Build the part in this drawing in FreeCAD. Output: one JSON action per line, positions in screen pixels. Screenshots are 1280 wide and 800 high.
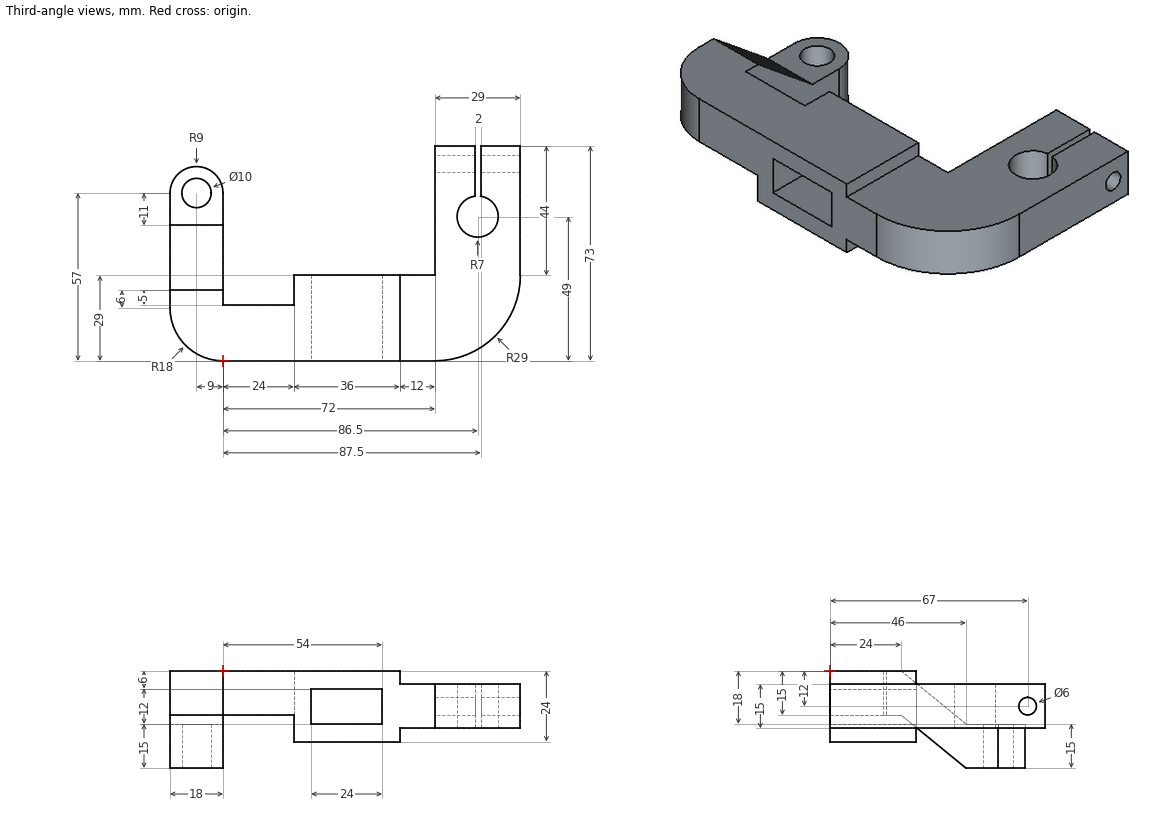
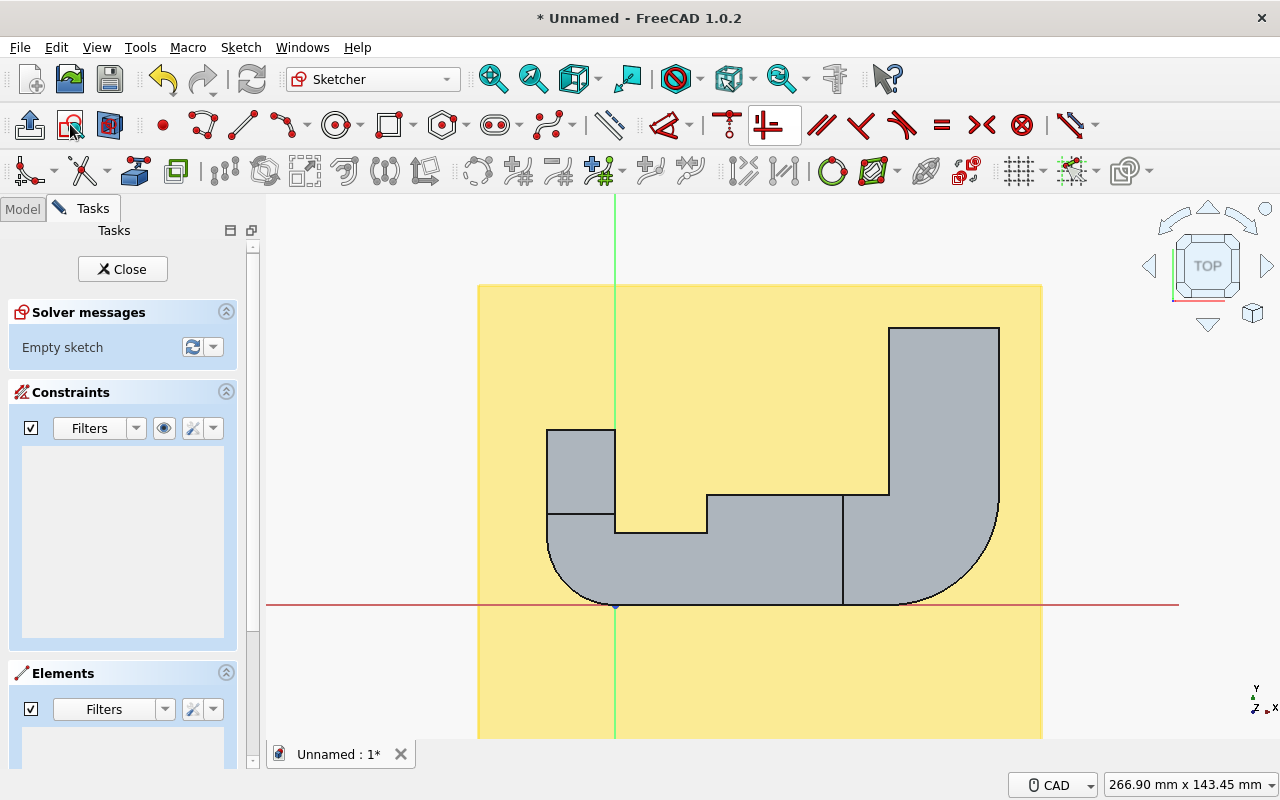
{"action": "left_click", "coordinate": [110, 126]}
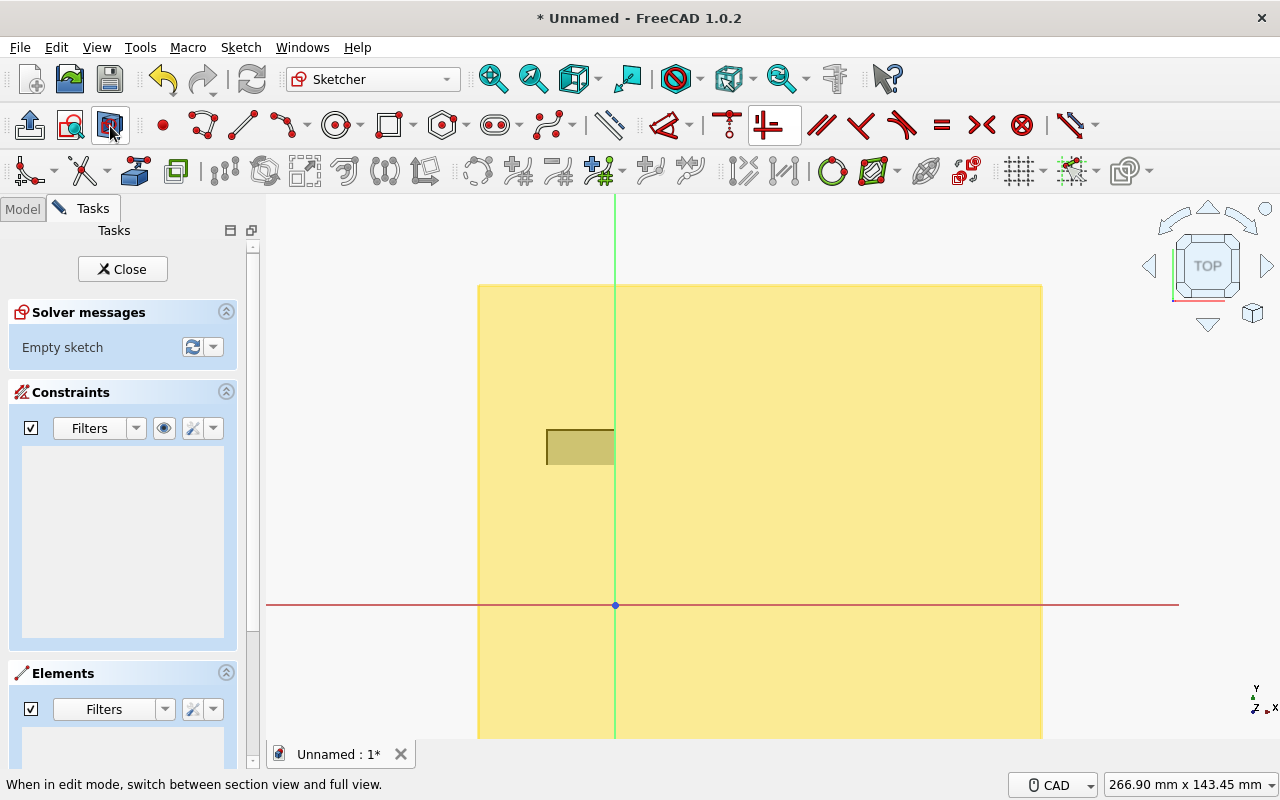
{"action": "scroll", "coordinate": [550, 374], "scroll_direction": "up", "scroll_amount": 8}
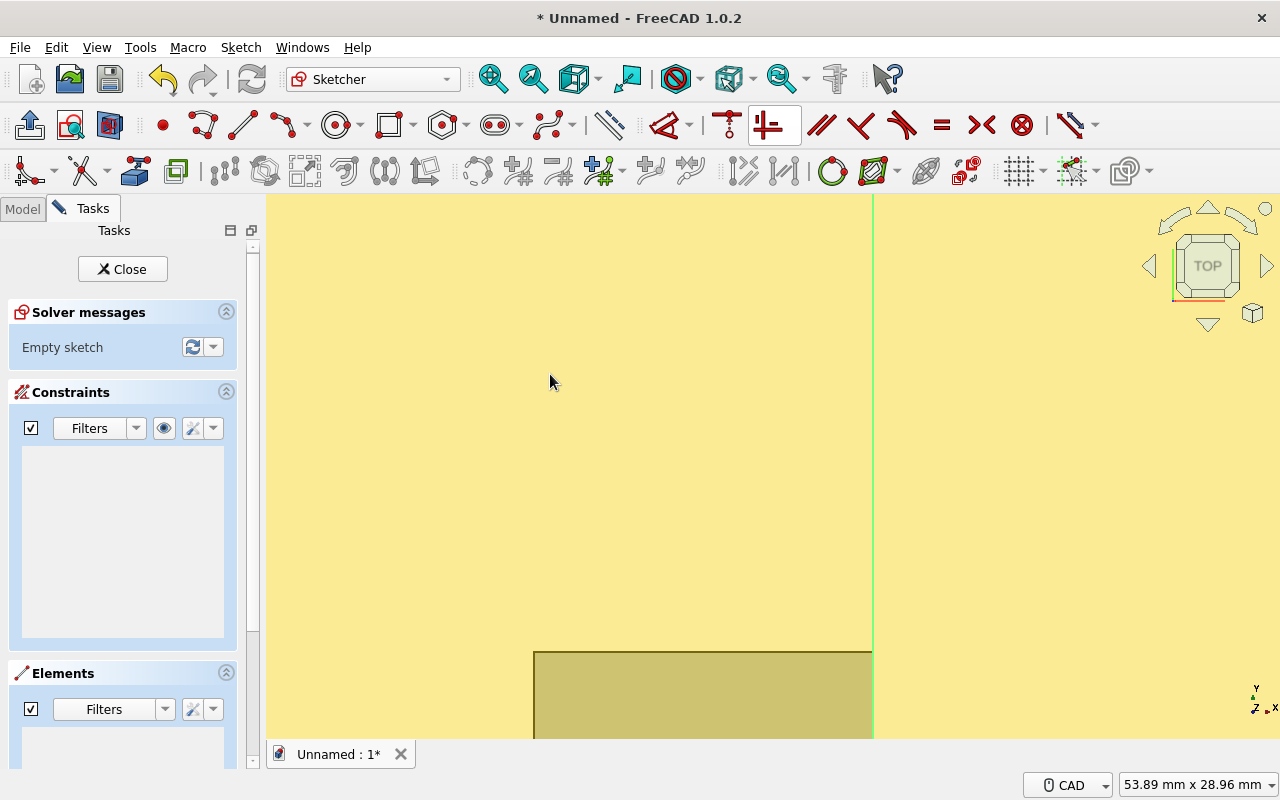
{"action": "left_click", "coordinate": [204, 126]}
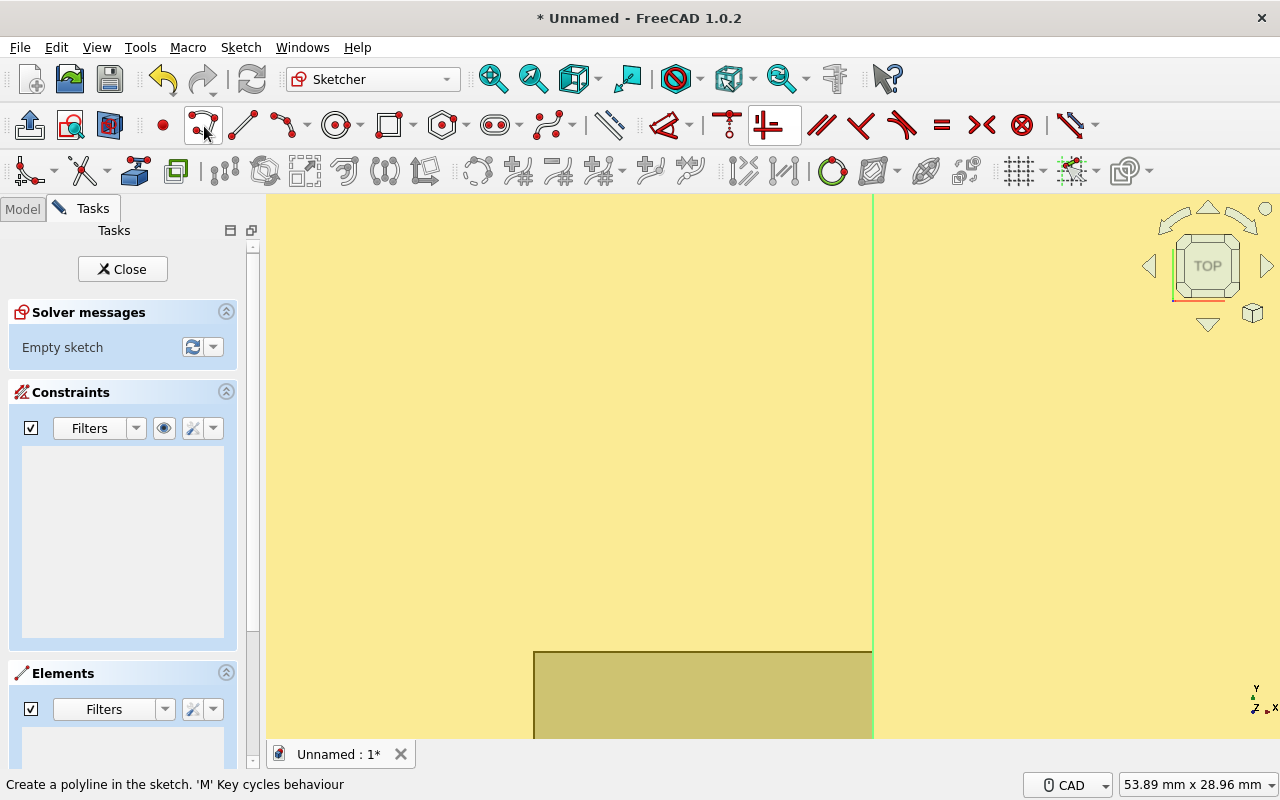
{"action": "left_click", "coordinate": [534, 445]}
{"action": "left_click", "coordinate": [534, 652]}
{"action": "left_click", "coordinate": [873, 652]}
{"action": "left_click", "coordinate": [864, 445]}
{"action": "right_click", "coordinate": [864, 445]}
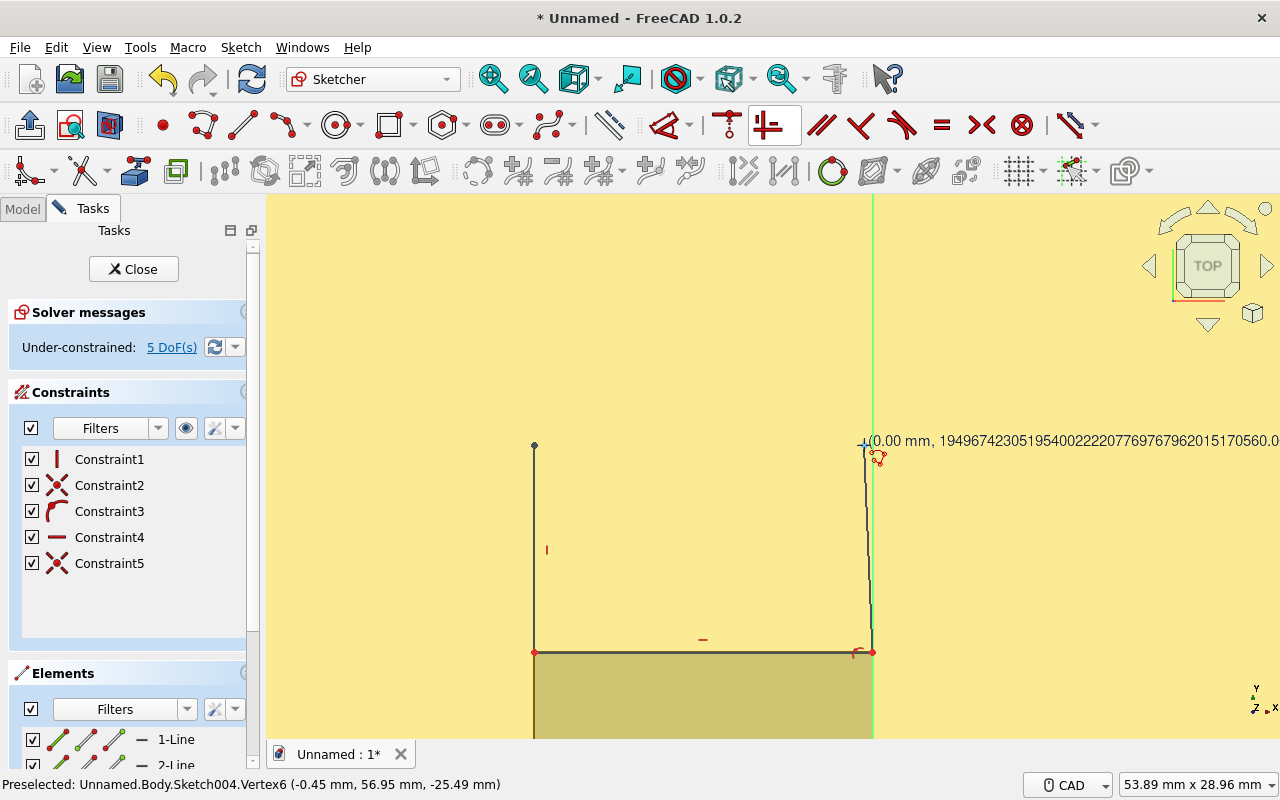
{"action": "left_click", "coordinate": [284, 126]}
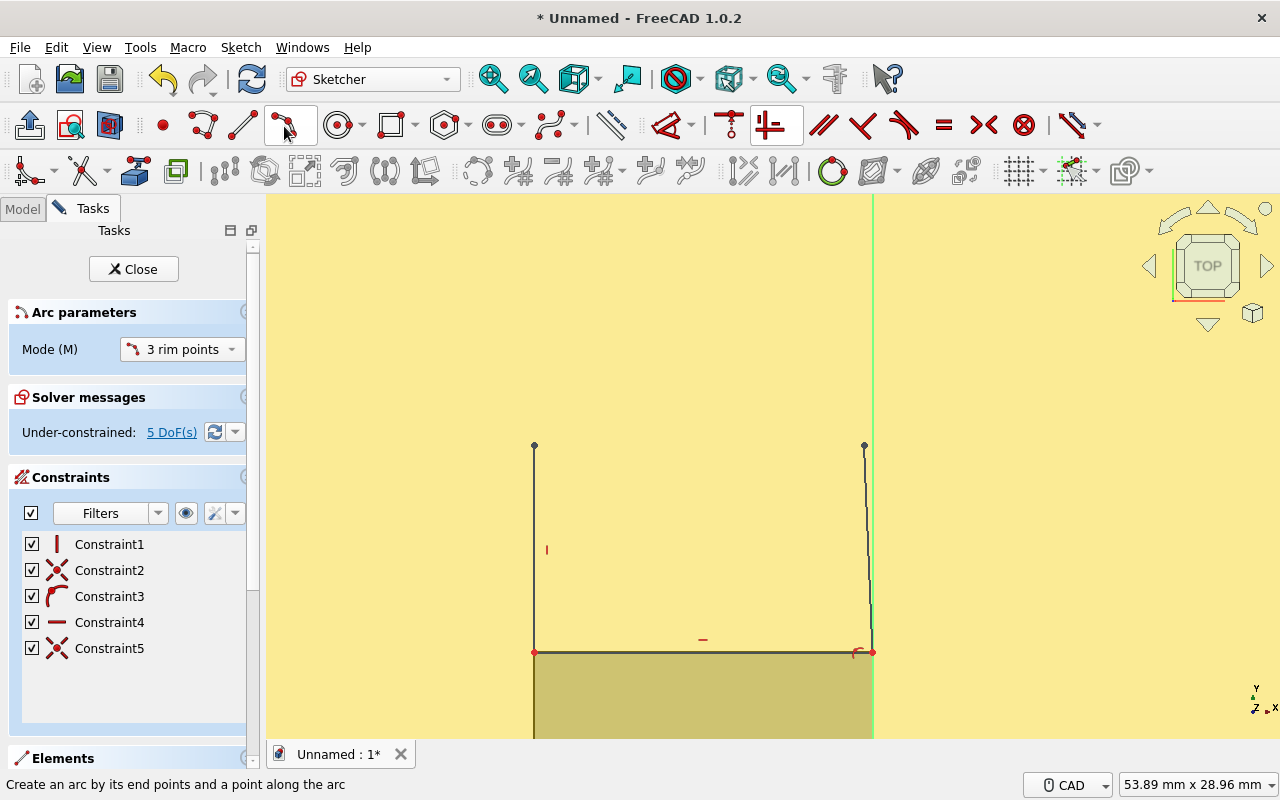
{"action": "left_click", "coordinate": [864, 446]}
{"action": "left_click", "coordinate": [534, 446]}
{"action": "left_click", "coordinate": [703, 276]}
{"action": "key", "text": "Escape"}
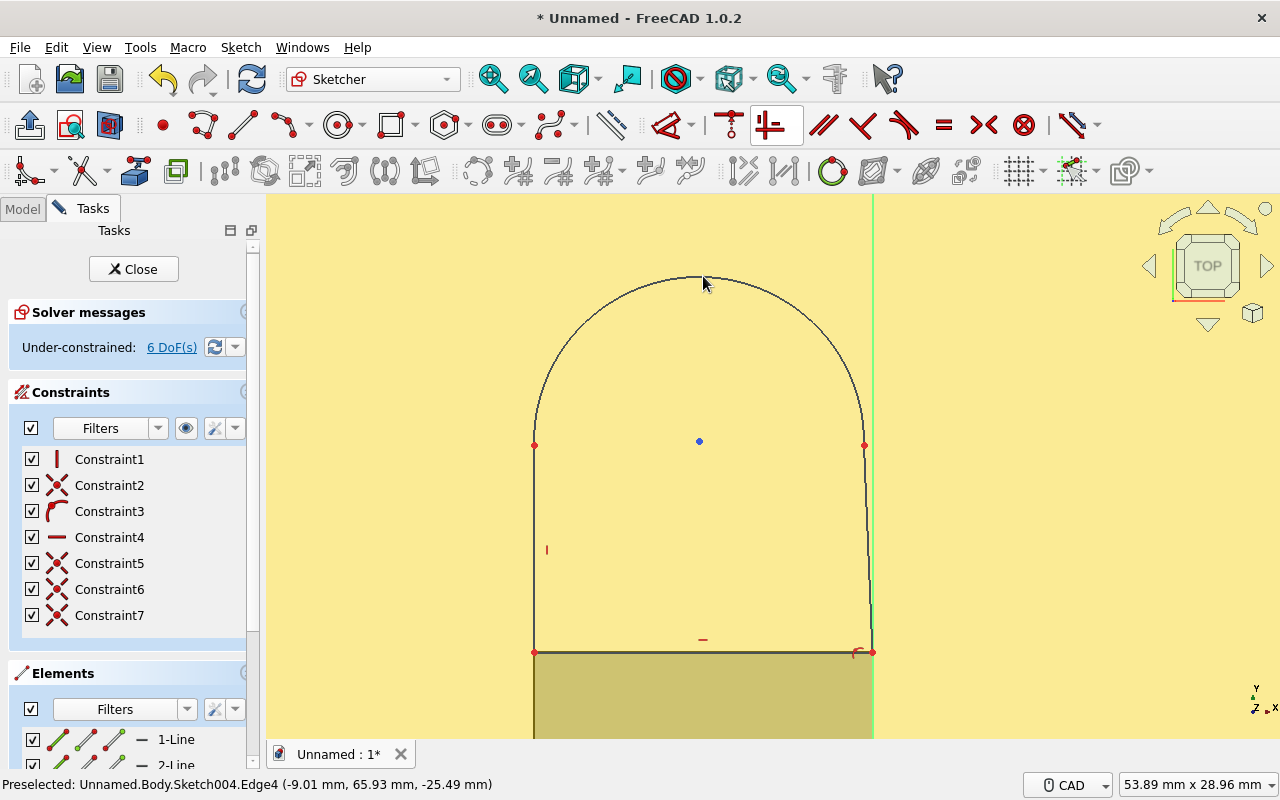
{"action": "left_click", "coordinate": [534, 508]}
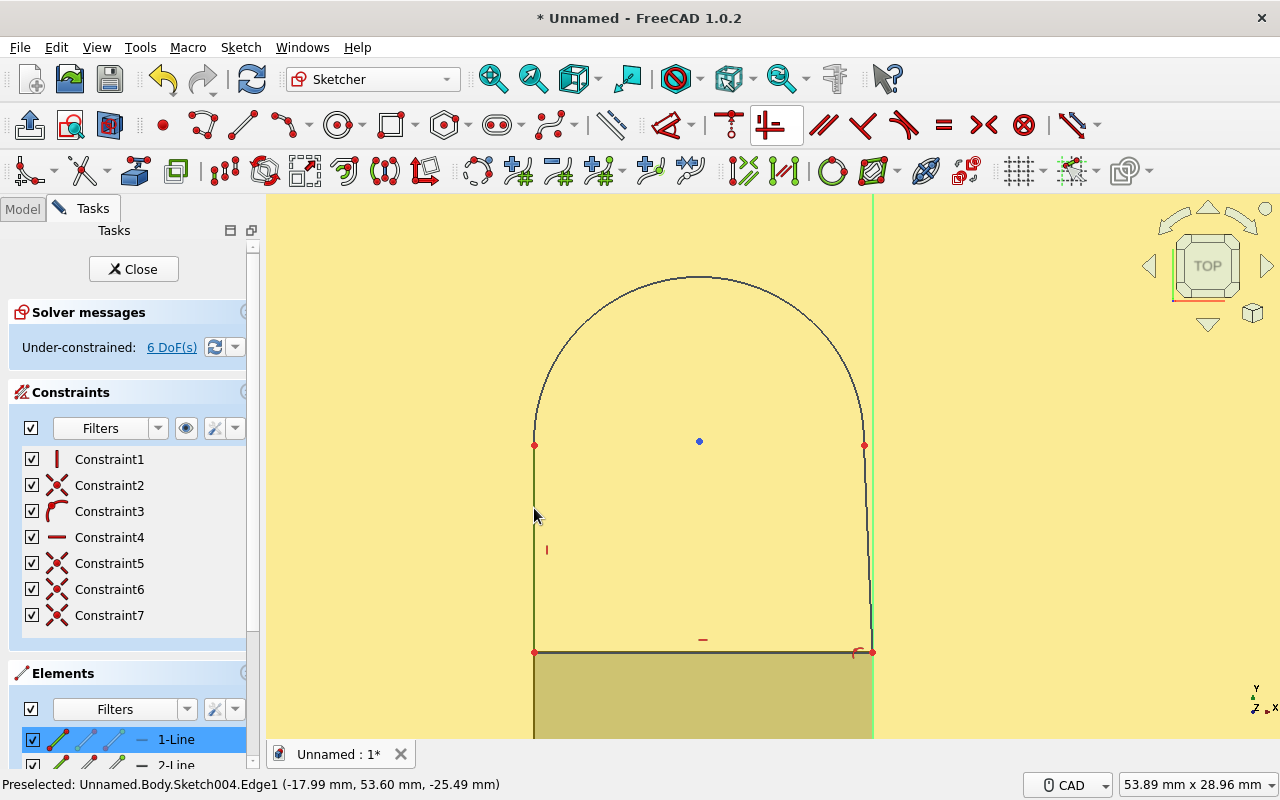
{"action": "left_click", "coordinate": [797, 309]}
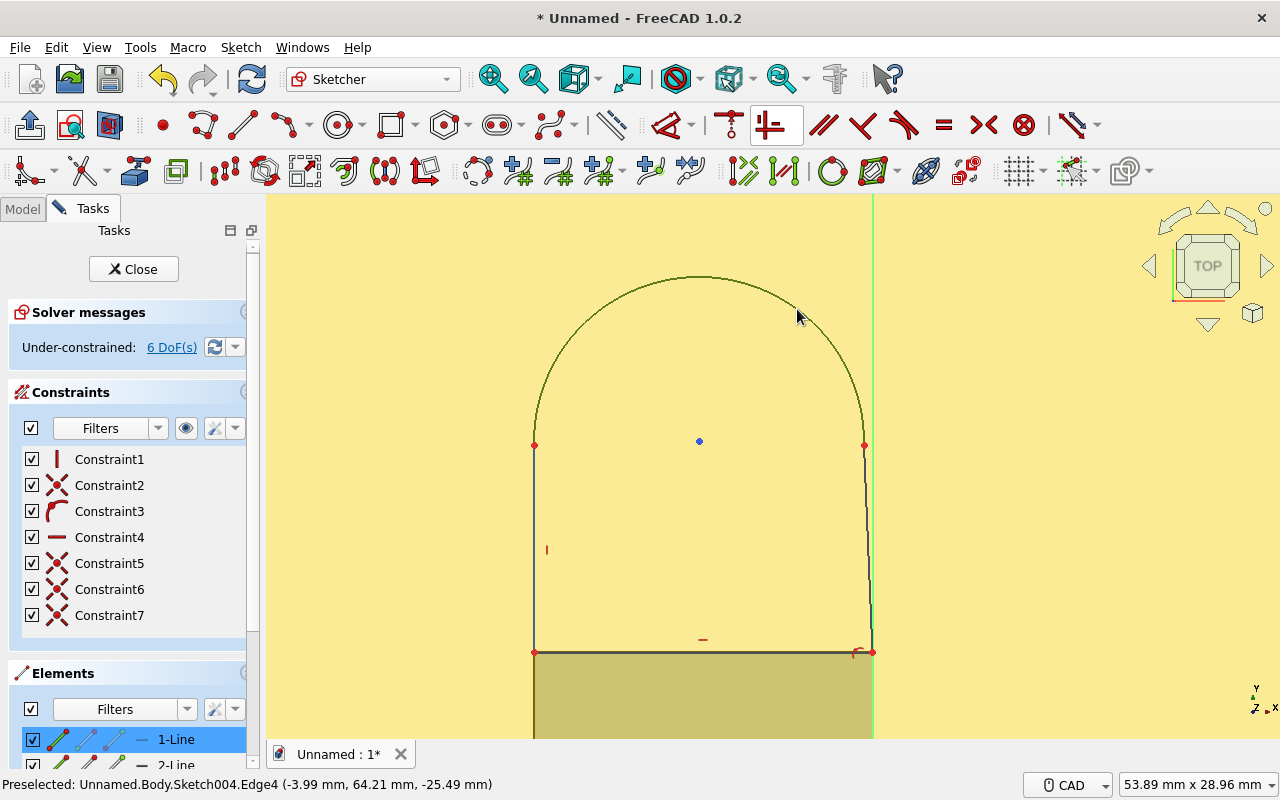
{"action": "left_click", "coordinate": [904, 126]}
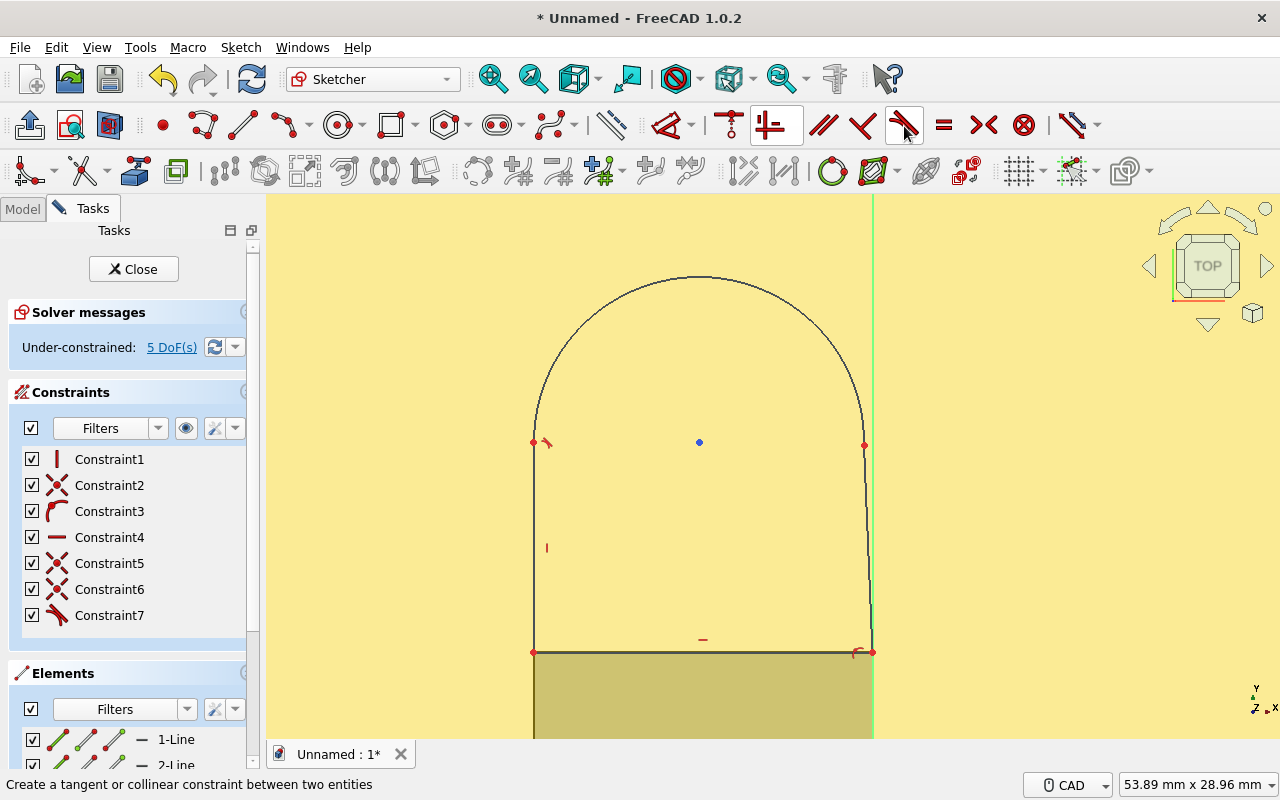
{"action": "left_click", "coordinate": [870, 591]}